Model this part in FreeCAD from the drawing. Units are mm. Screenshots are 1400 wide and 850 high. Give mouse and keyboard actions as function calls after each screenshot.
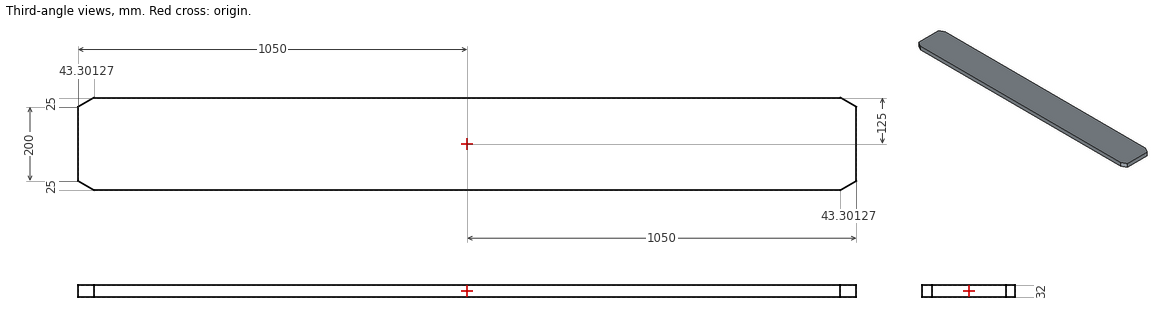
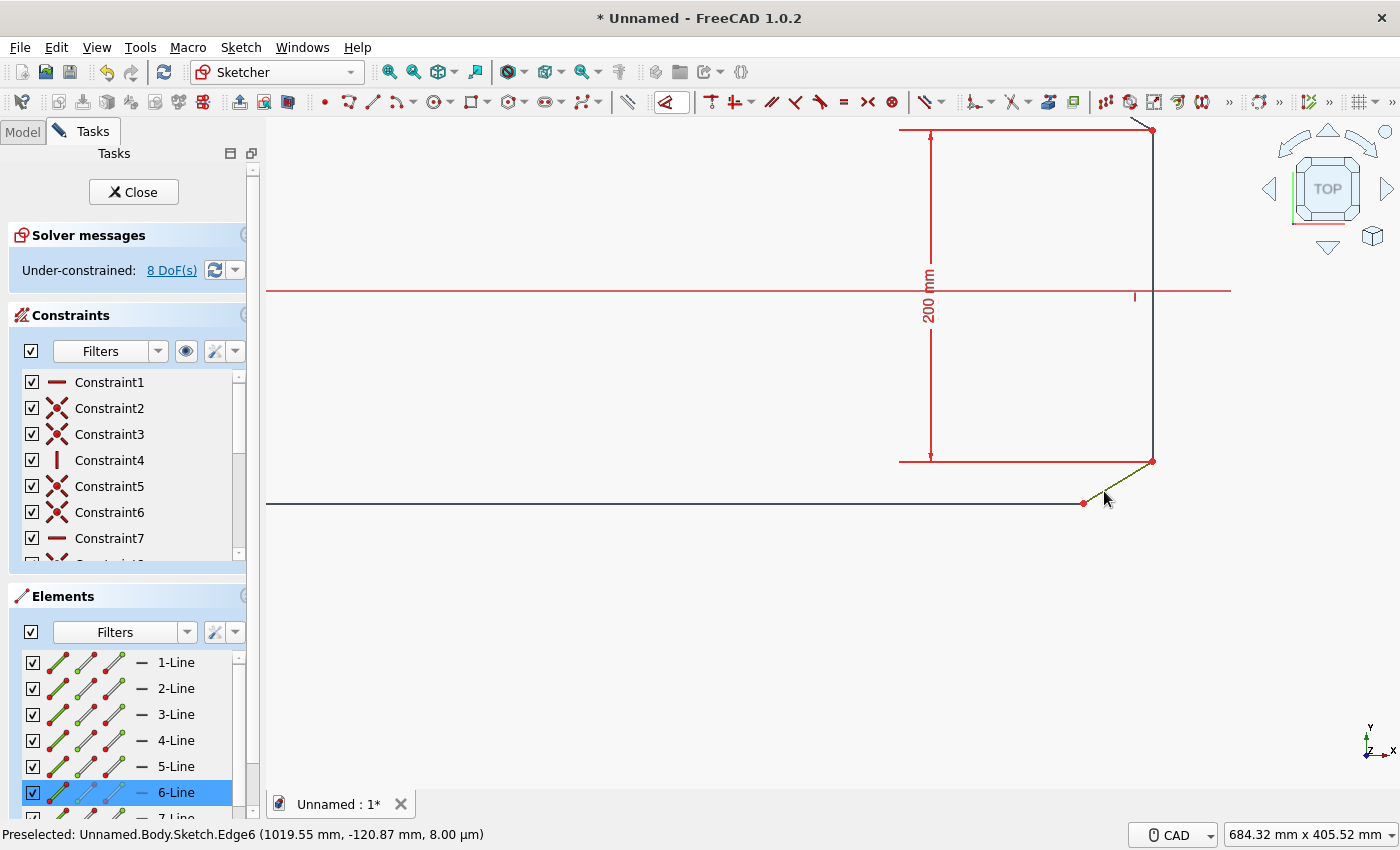
click(684, 102)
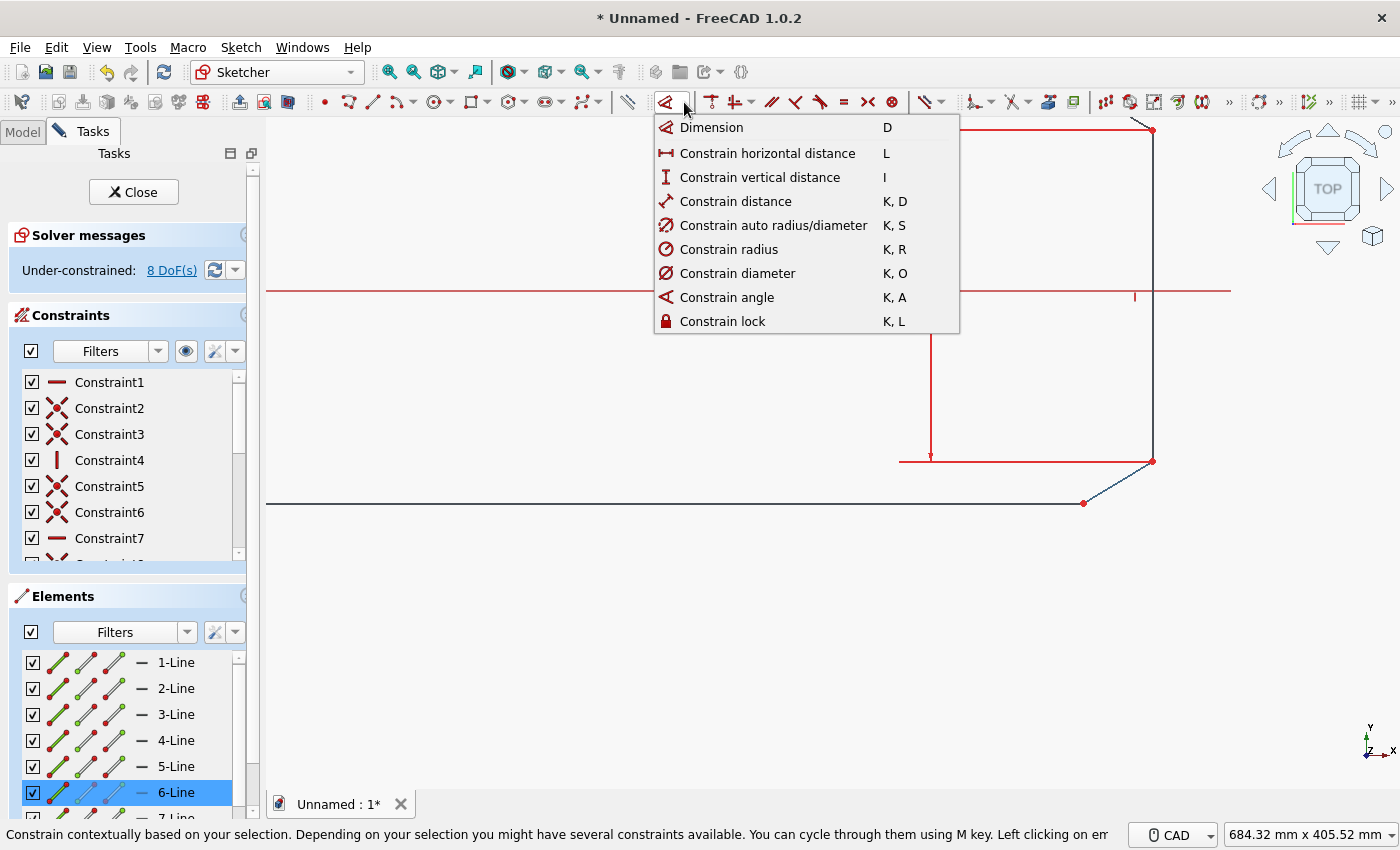
click(807, 177)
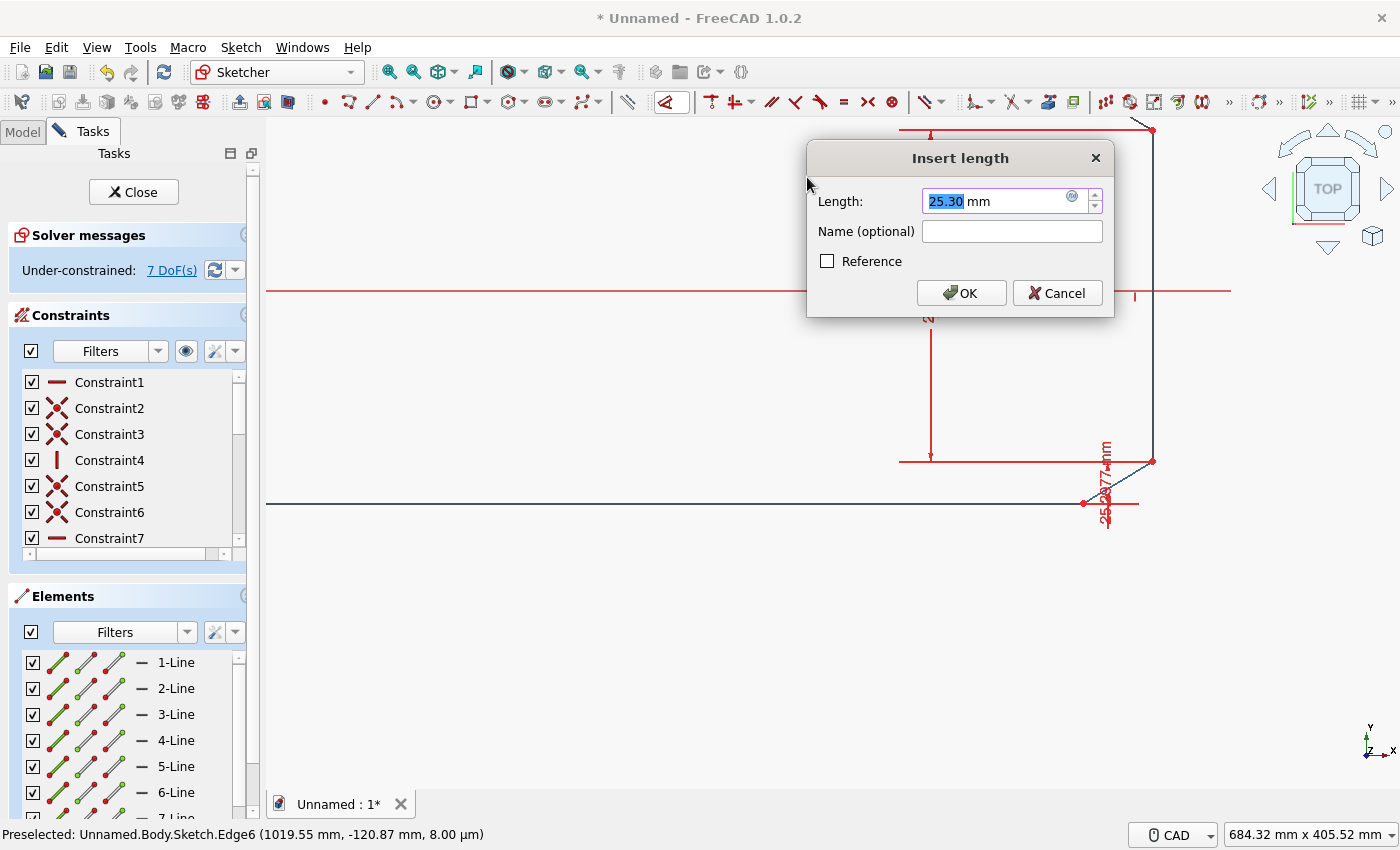
text(25)
key(Return)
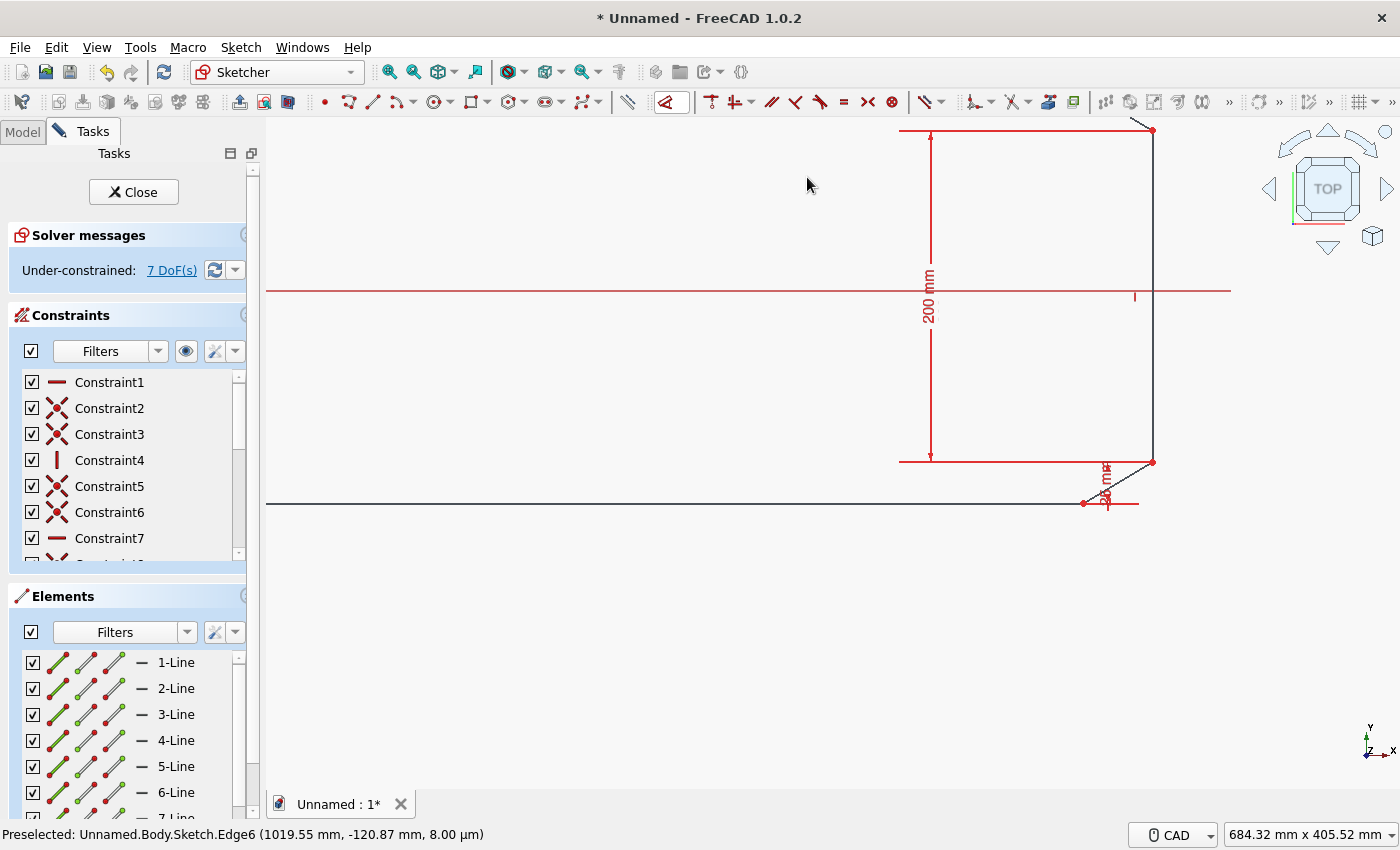
scroll(1106, 494, down, 8)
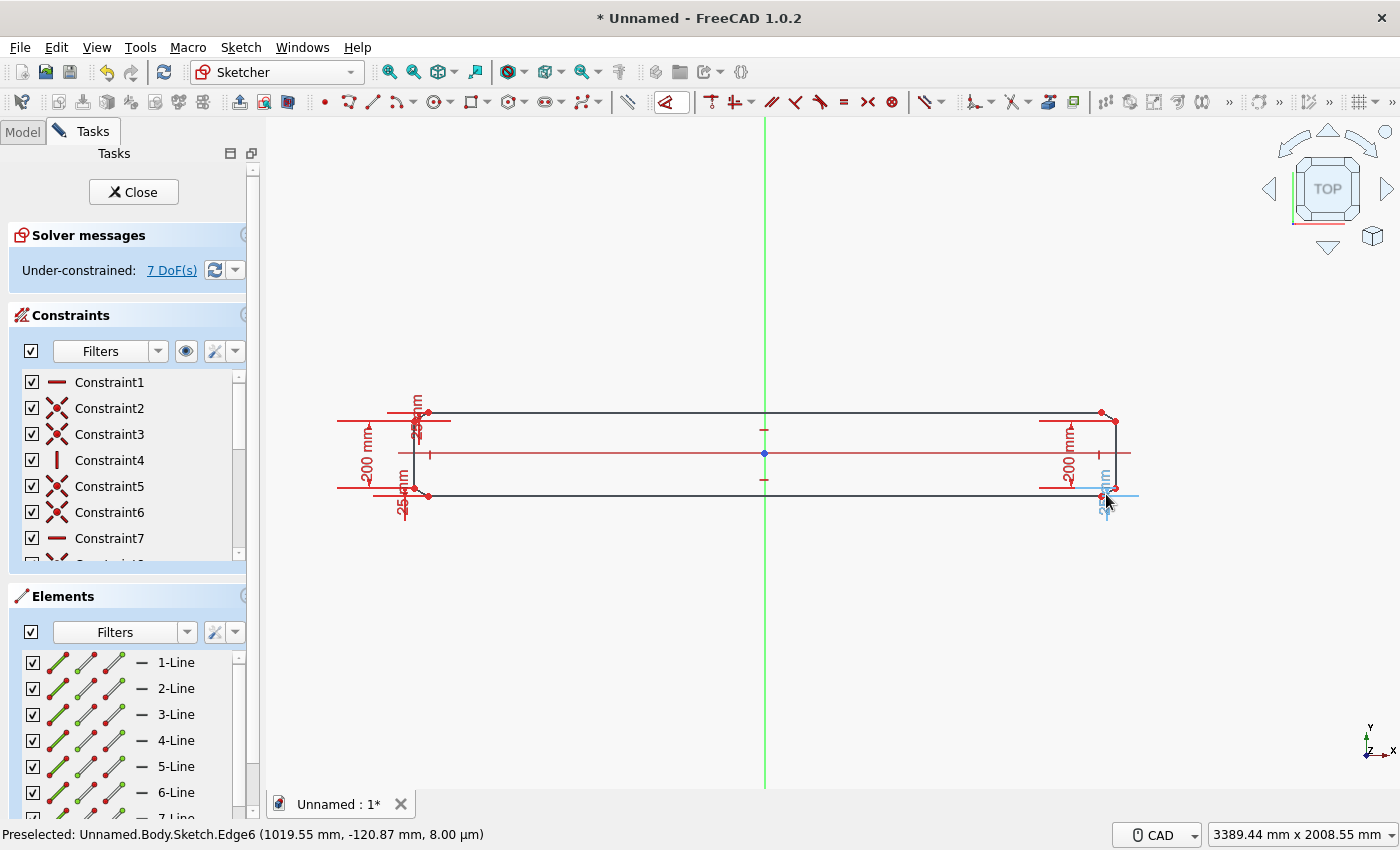
click(1102, 413)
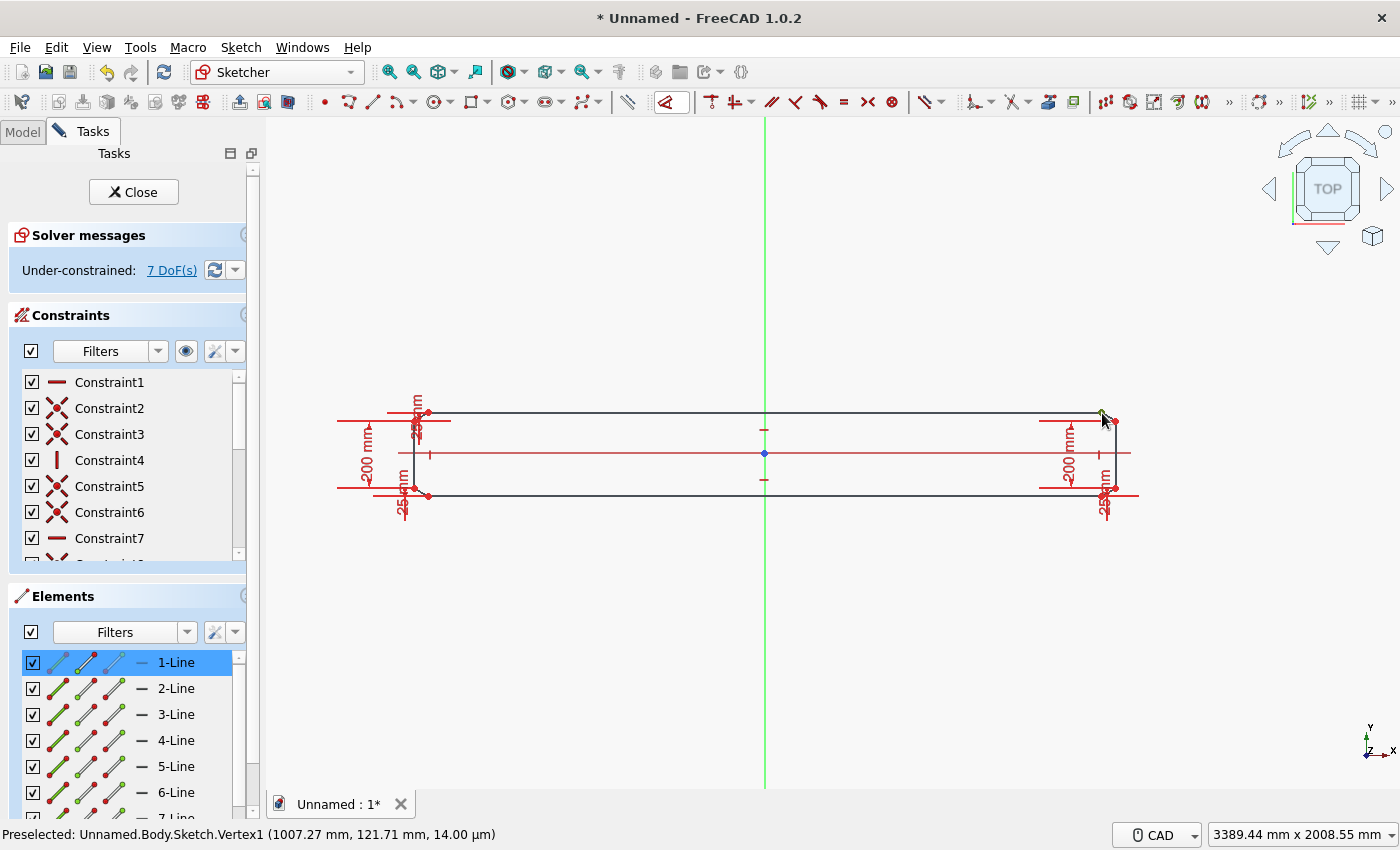
key(i)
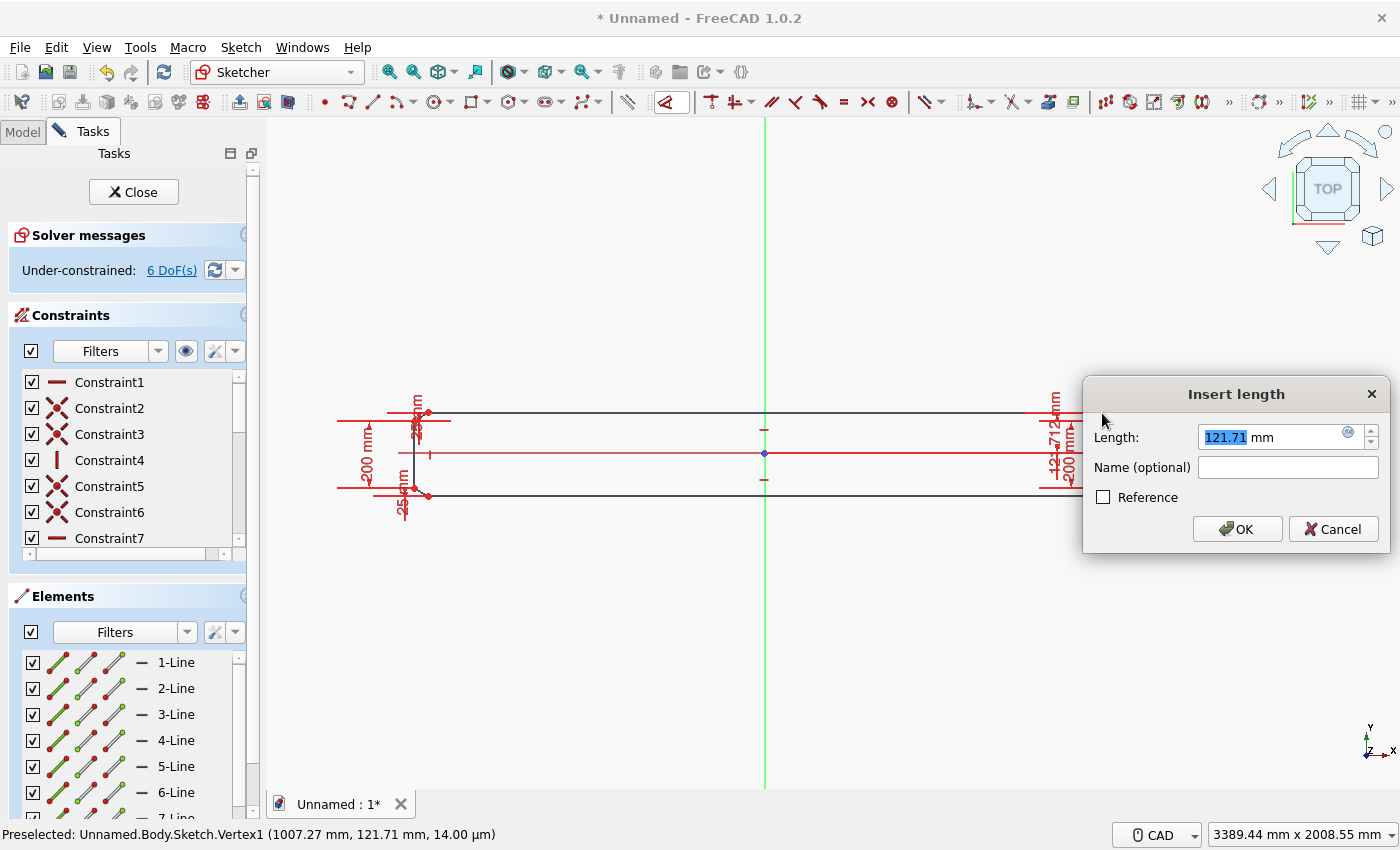
text(125)
key(Return)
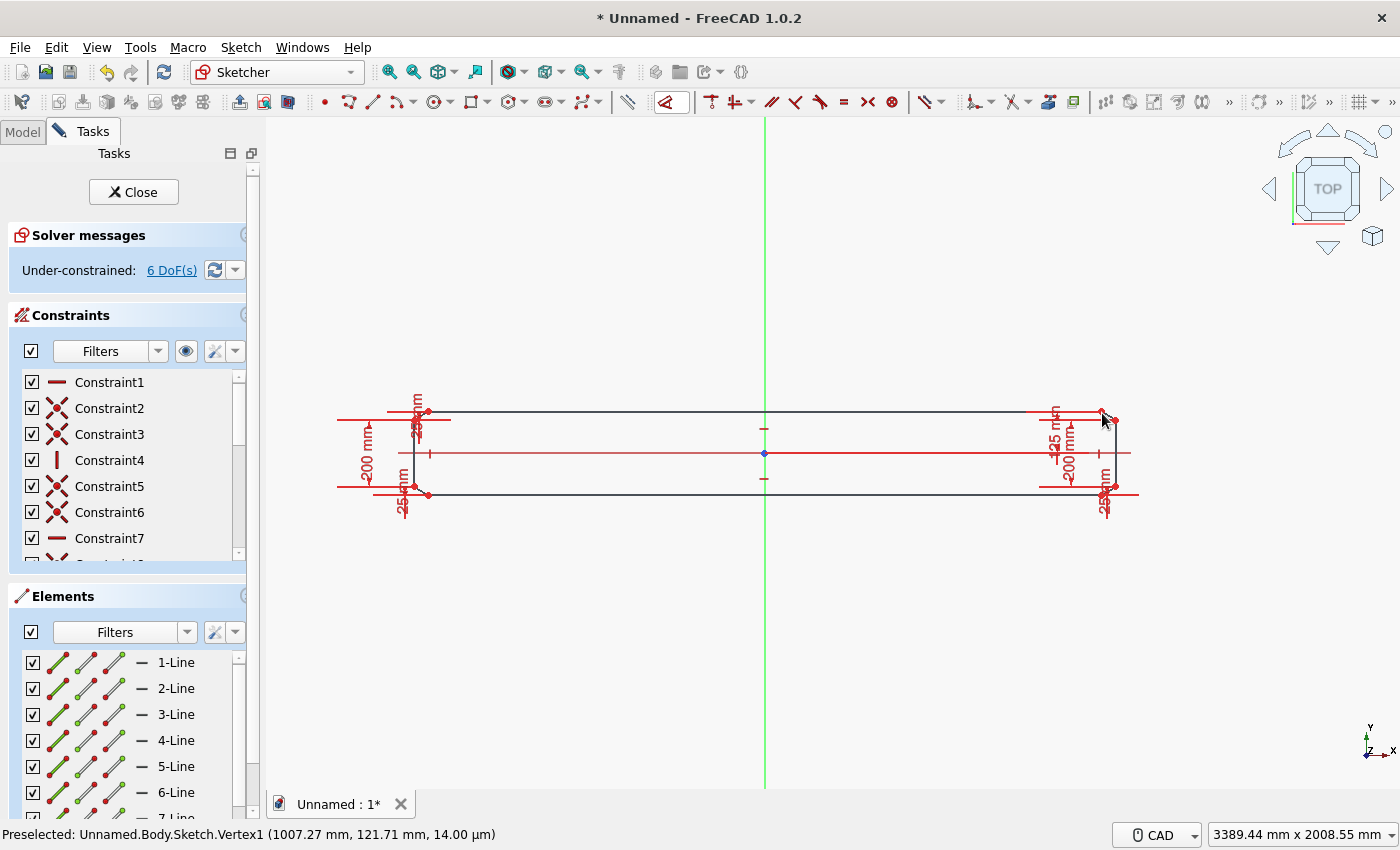
click(414, 420)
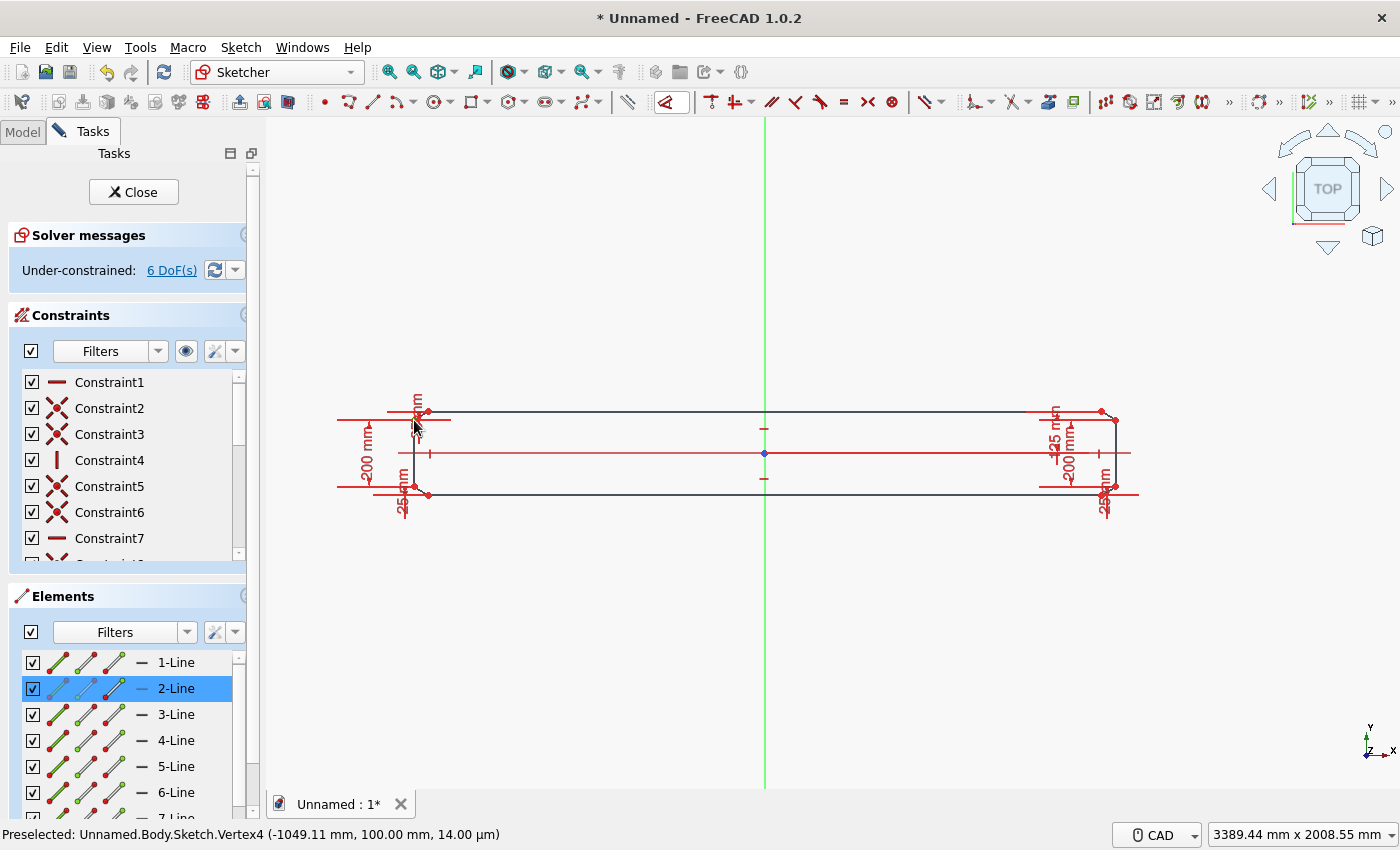
click(684, 102)